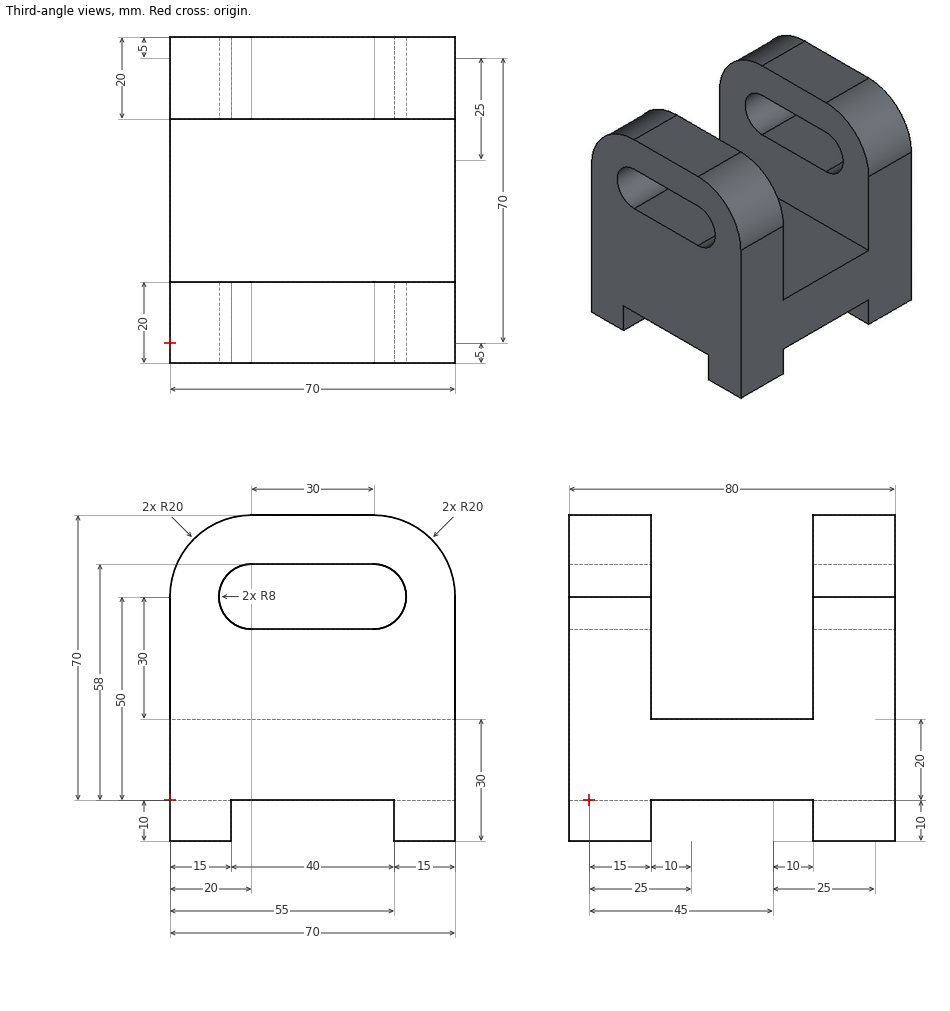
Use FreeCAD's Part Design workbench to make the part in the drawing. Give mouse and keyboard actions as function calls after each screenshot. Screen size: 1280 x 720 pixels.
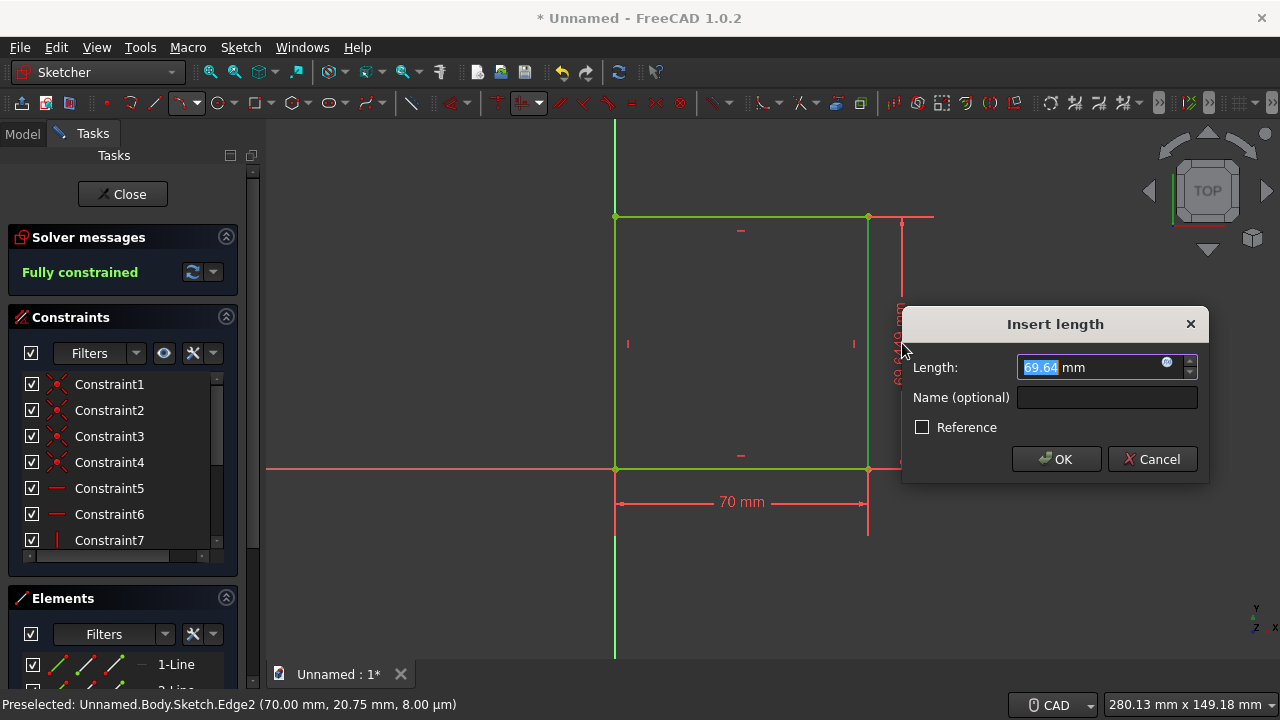
text(70)
key(Return)
key(Escape)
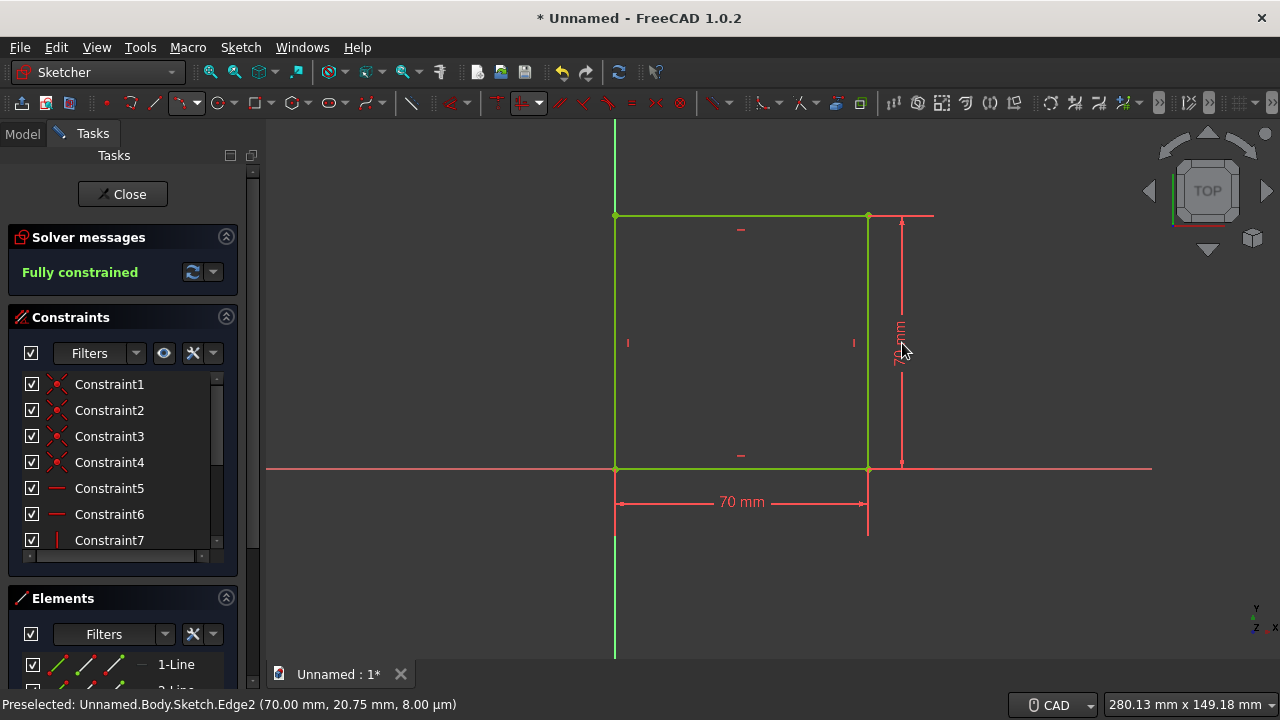
click(123, 194)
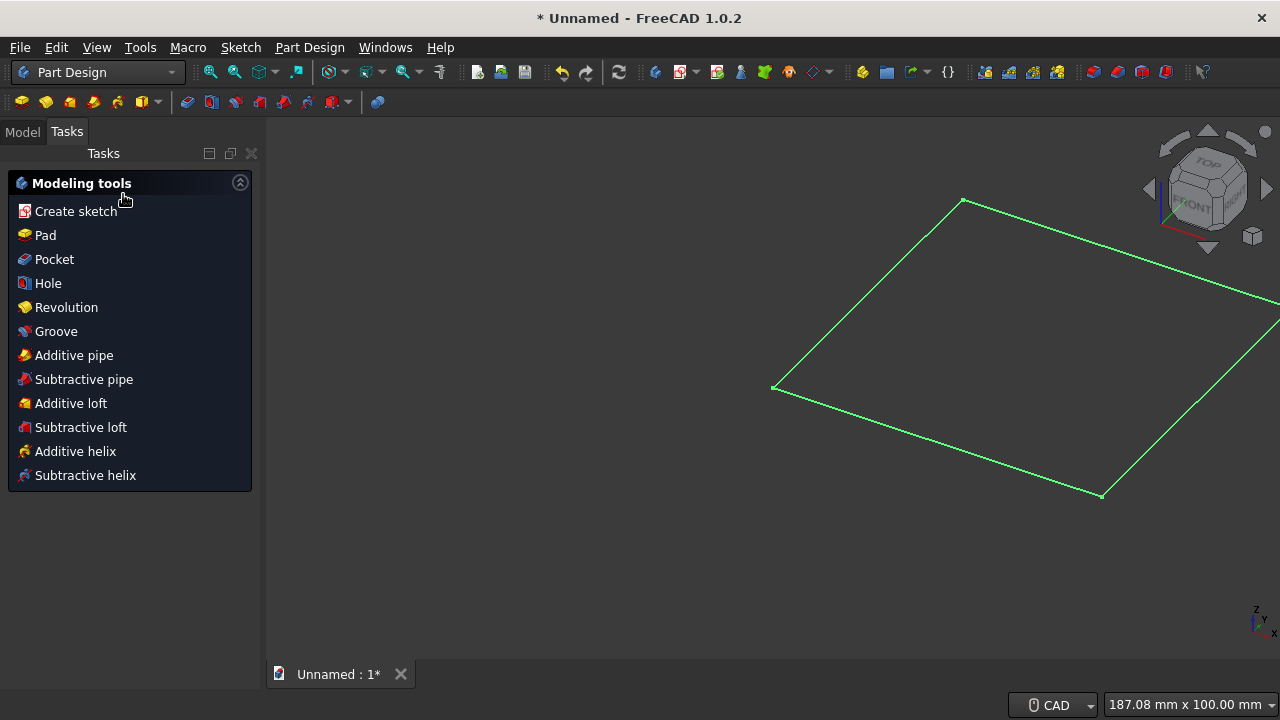
click(22, 102)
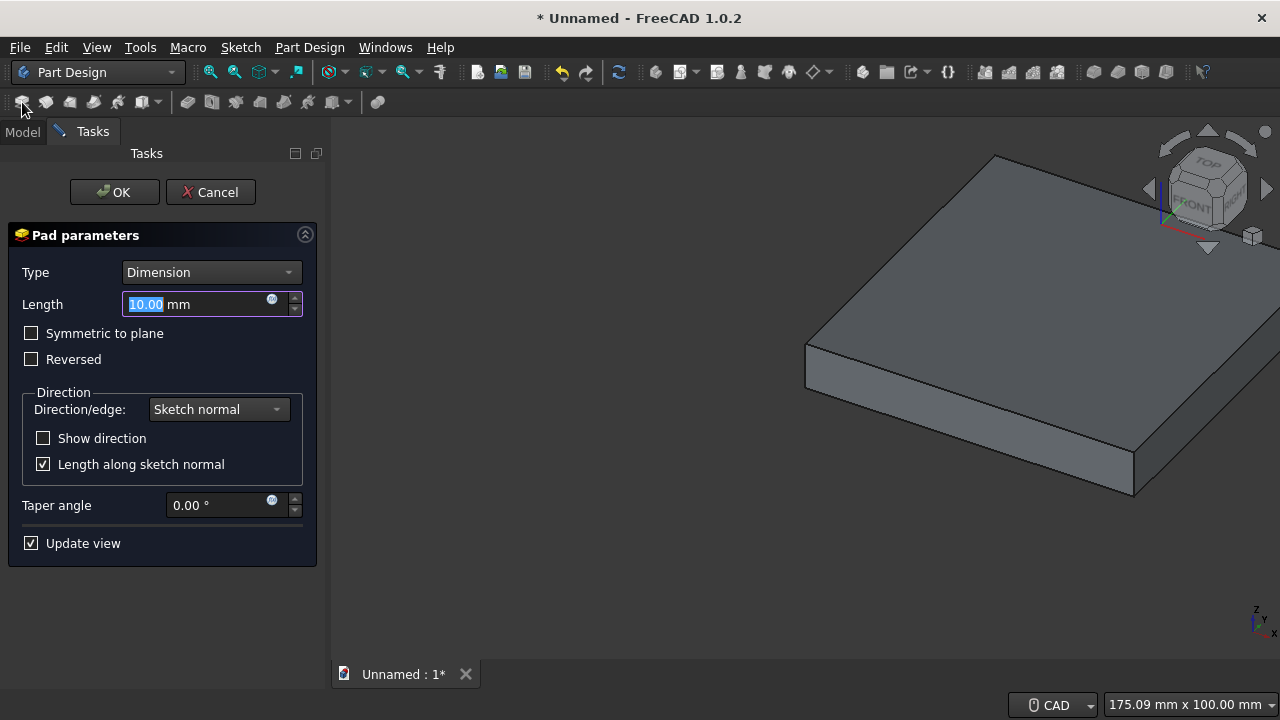
text(20)
key(Tab)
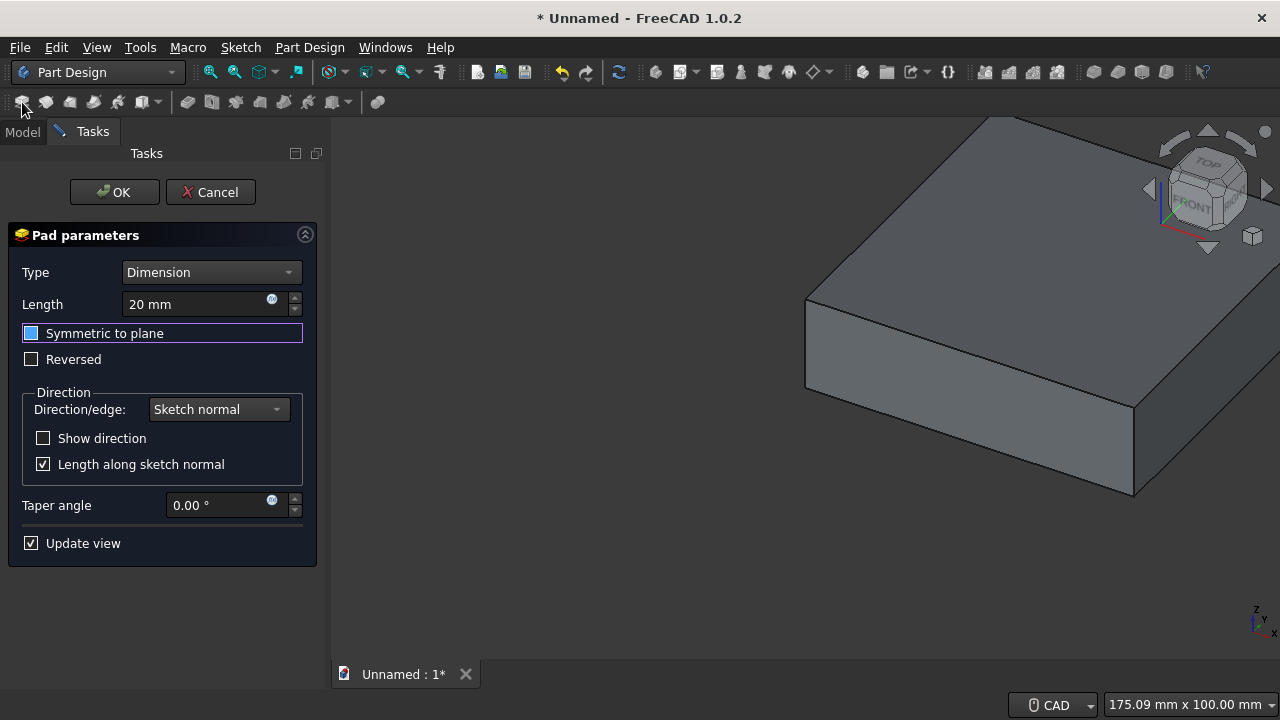
click(115, 192)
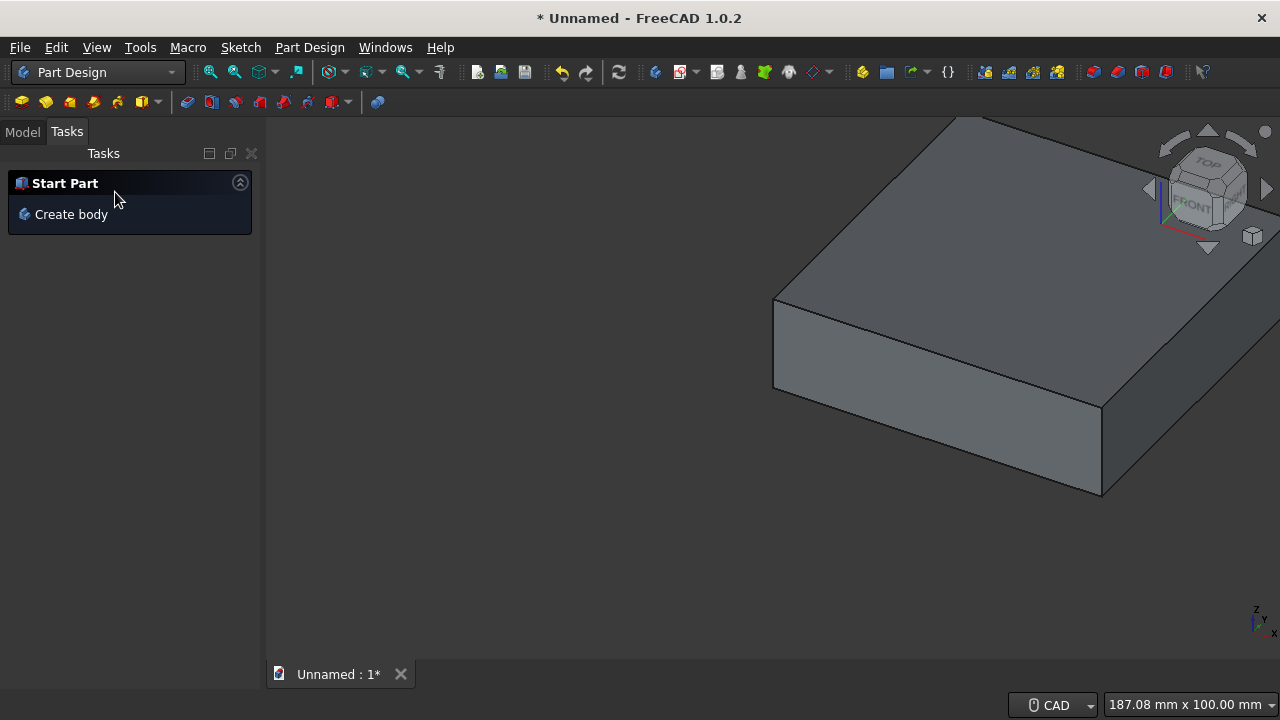
click(212, 72)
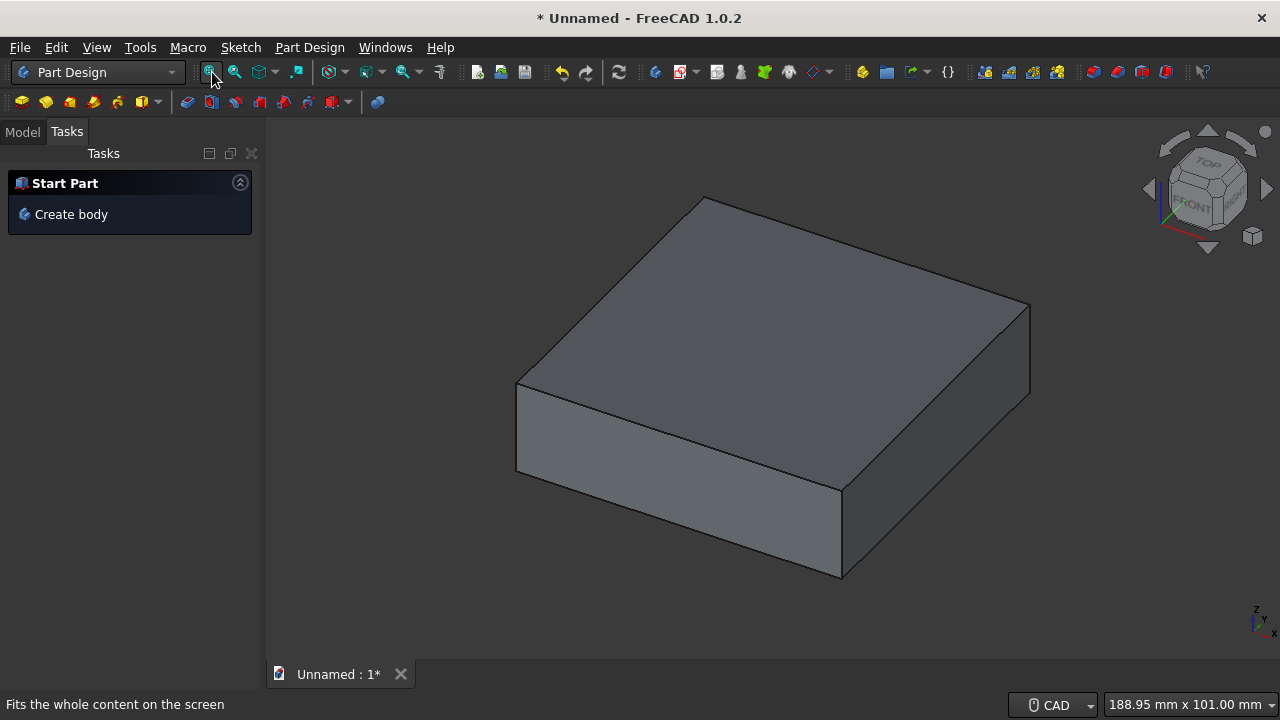
click(772, 511)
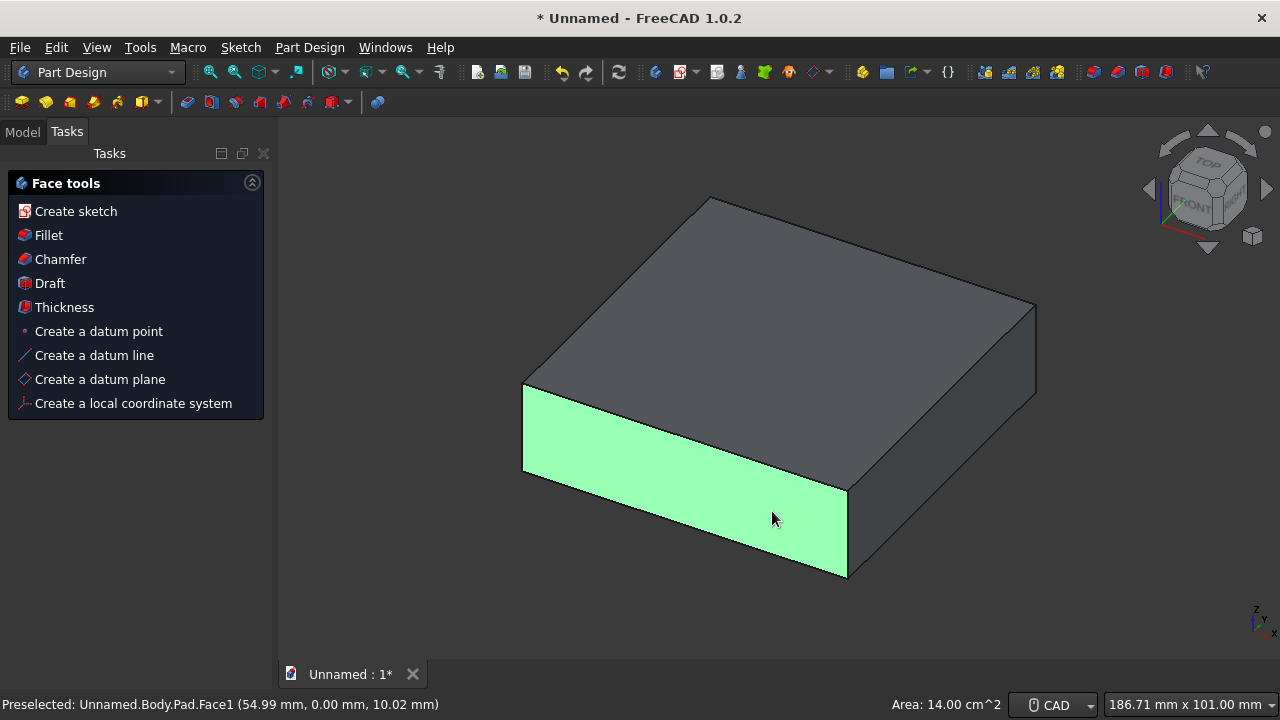
click(680, 72)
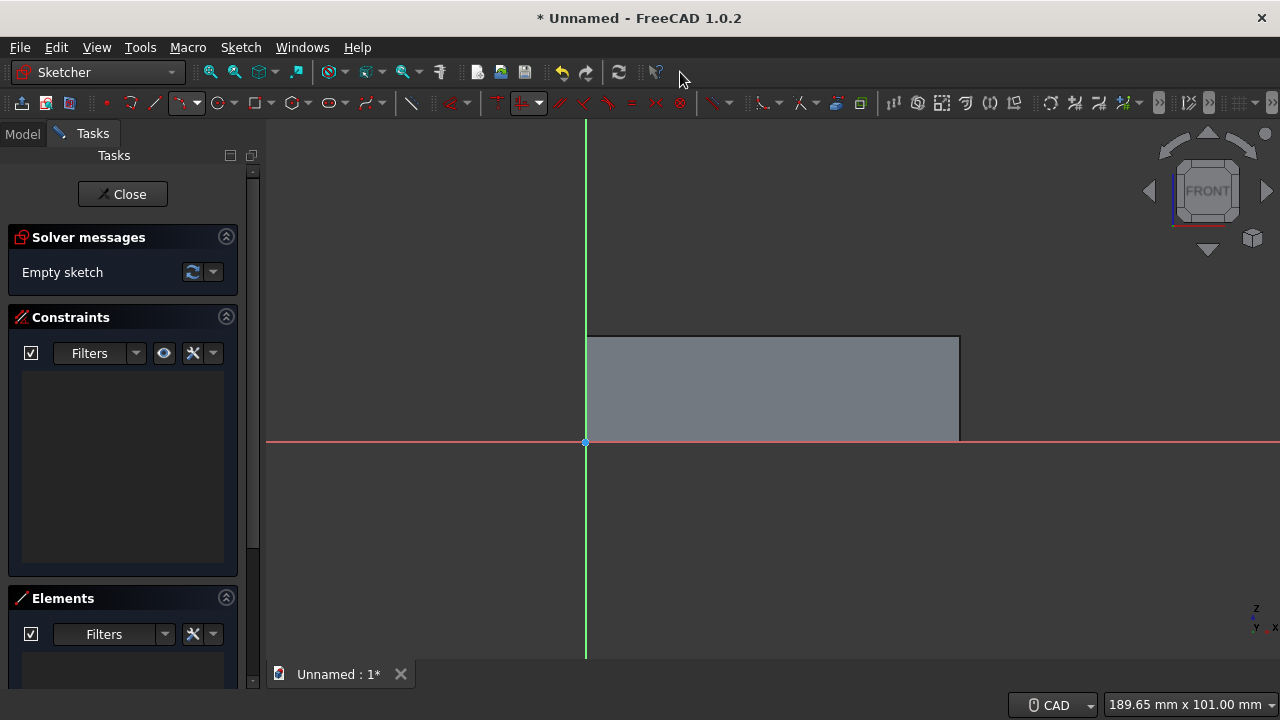
scroll(912, 631, up, 2)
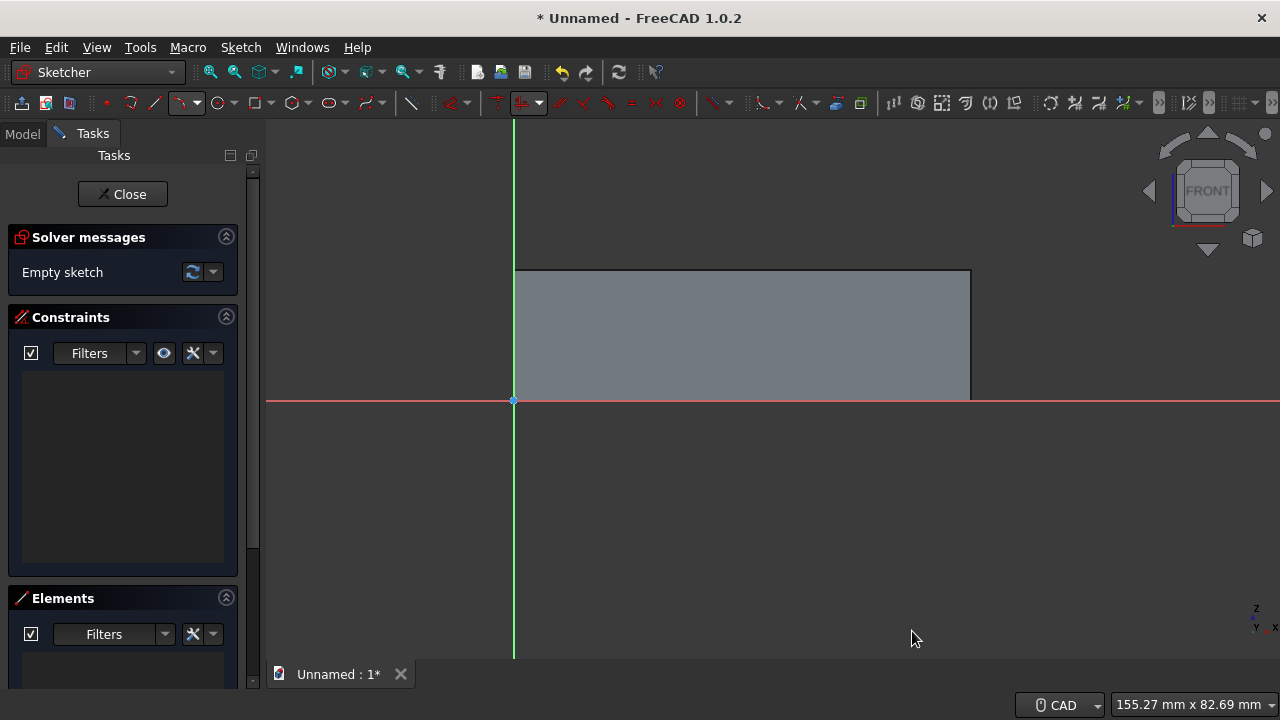
key(g)
key(r)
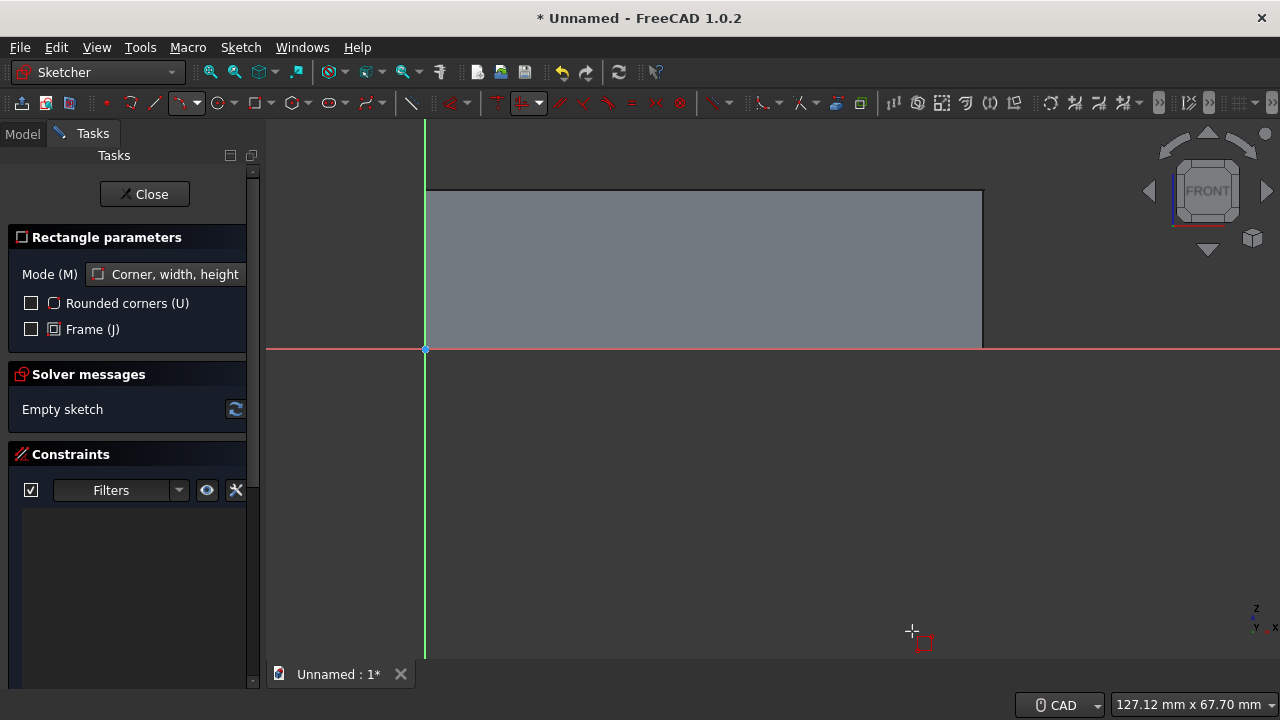
click(425, 349)
click(545, 429)